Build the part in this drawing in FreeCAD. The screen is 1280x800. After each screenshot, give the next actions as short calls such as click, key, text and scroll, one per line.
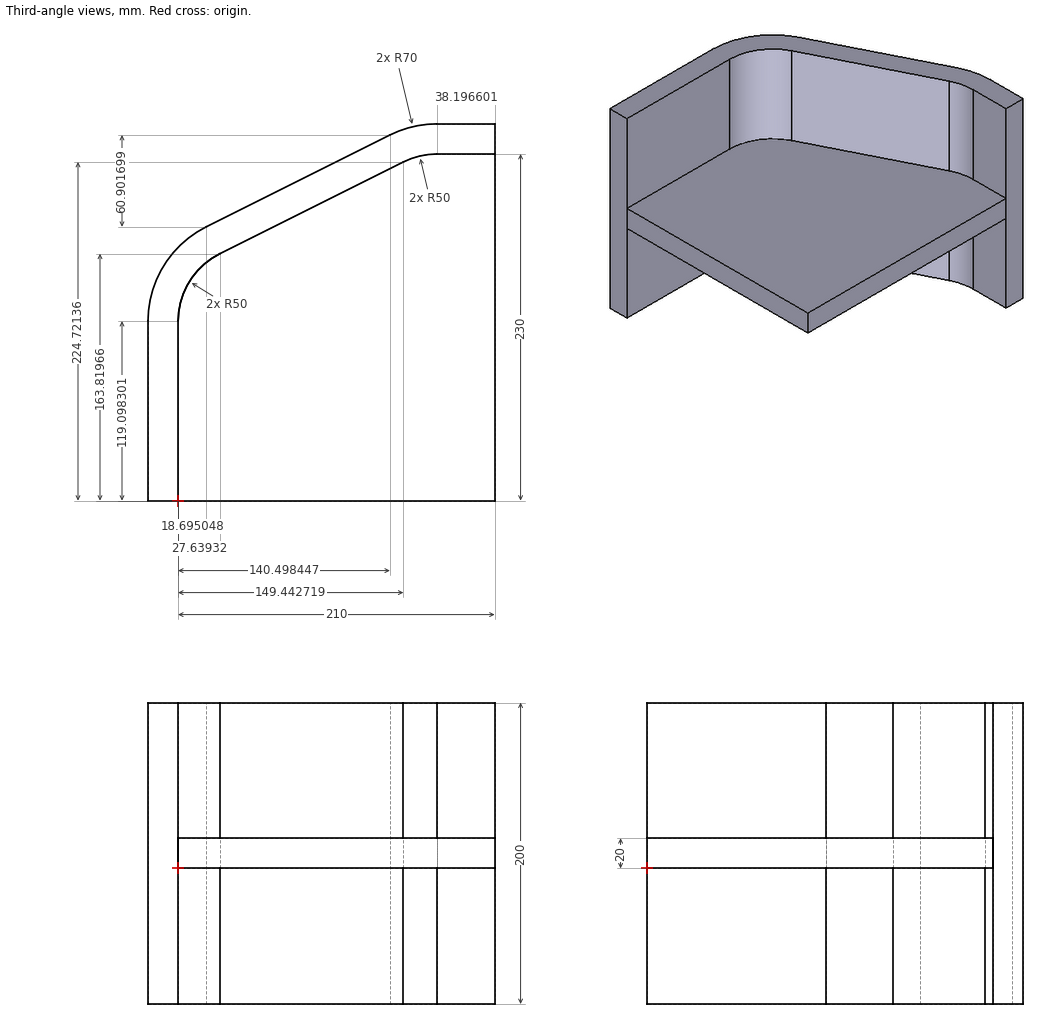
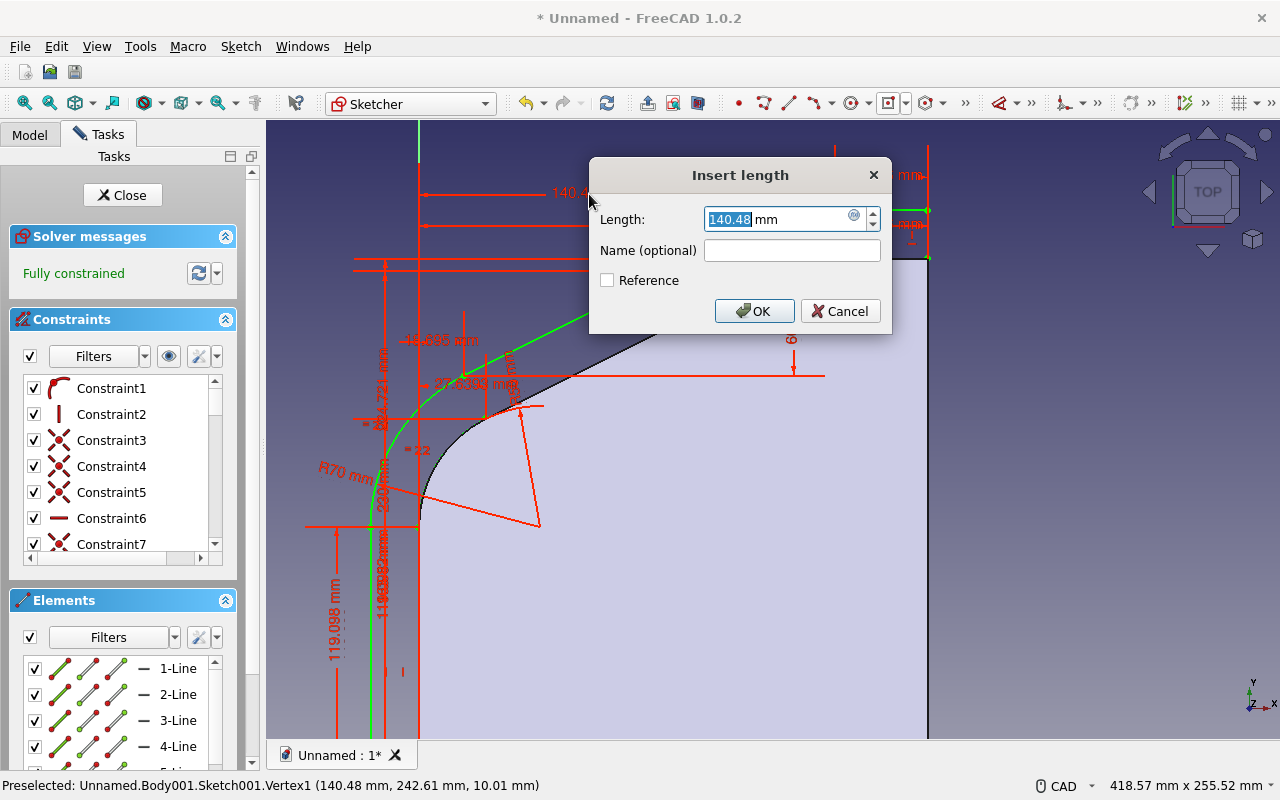
text(140.498447)
key(Return)
key(Escape)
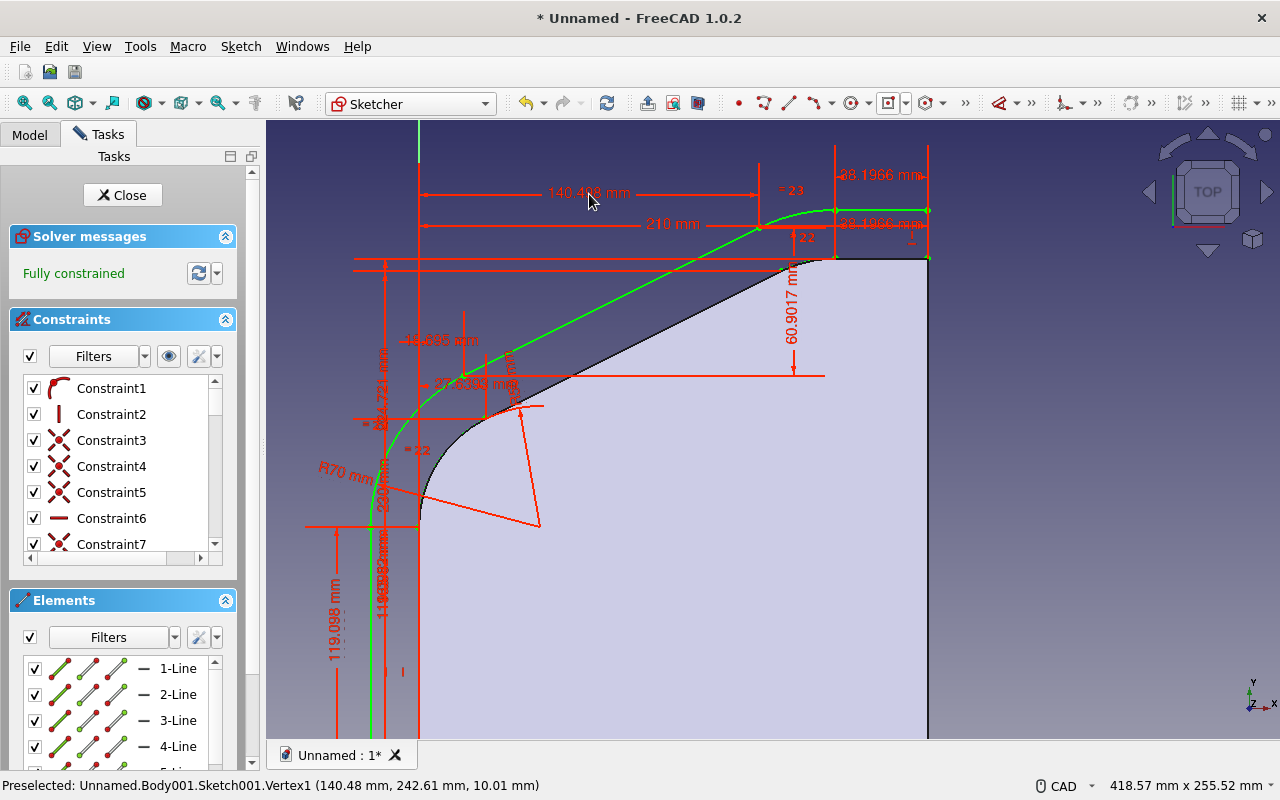
click(123, 195)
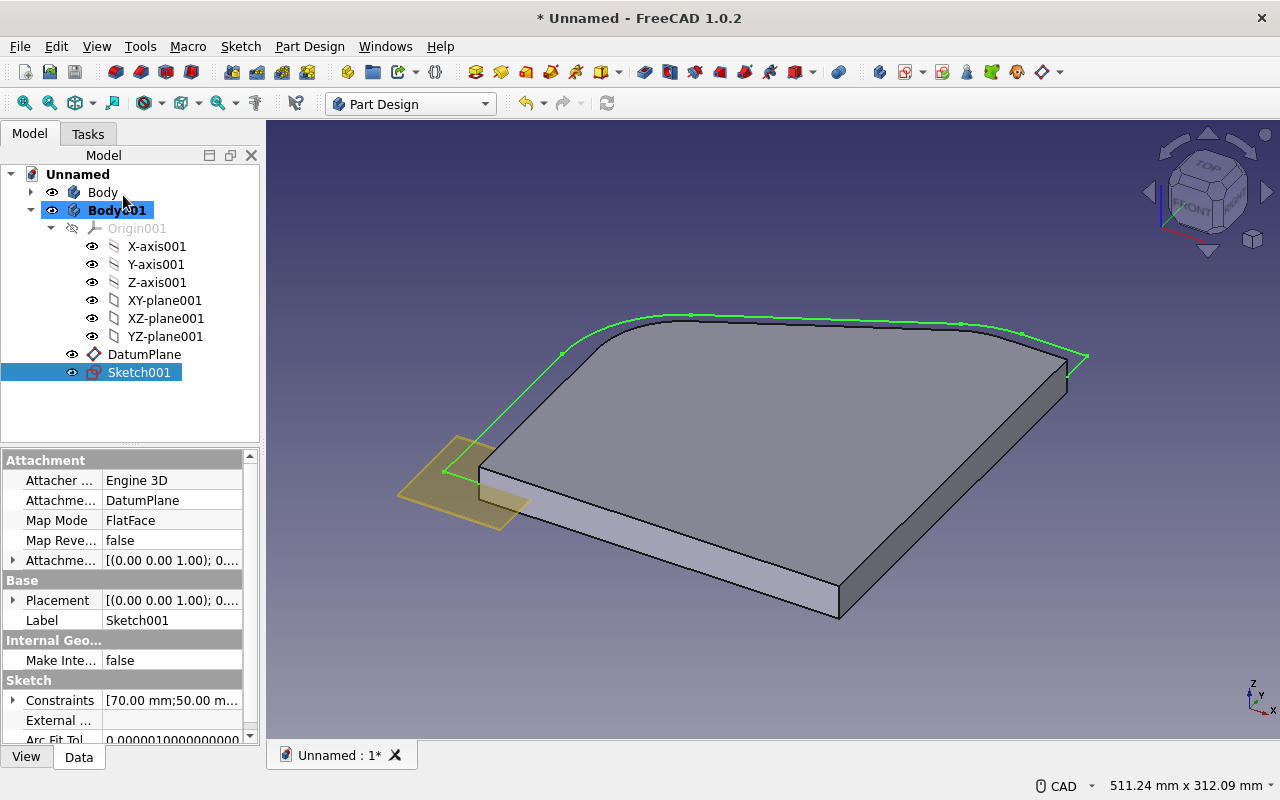
click(476, 72)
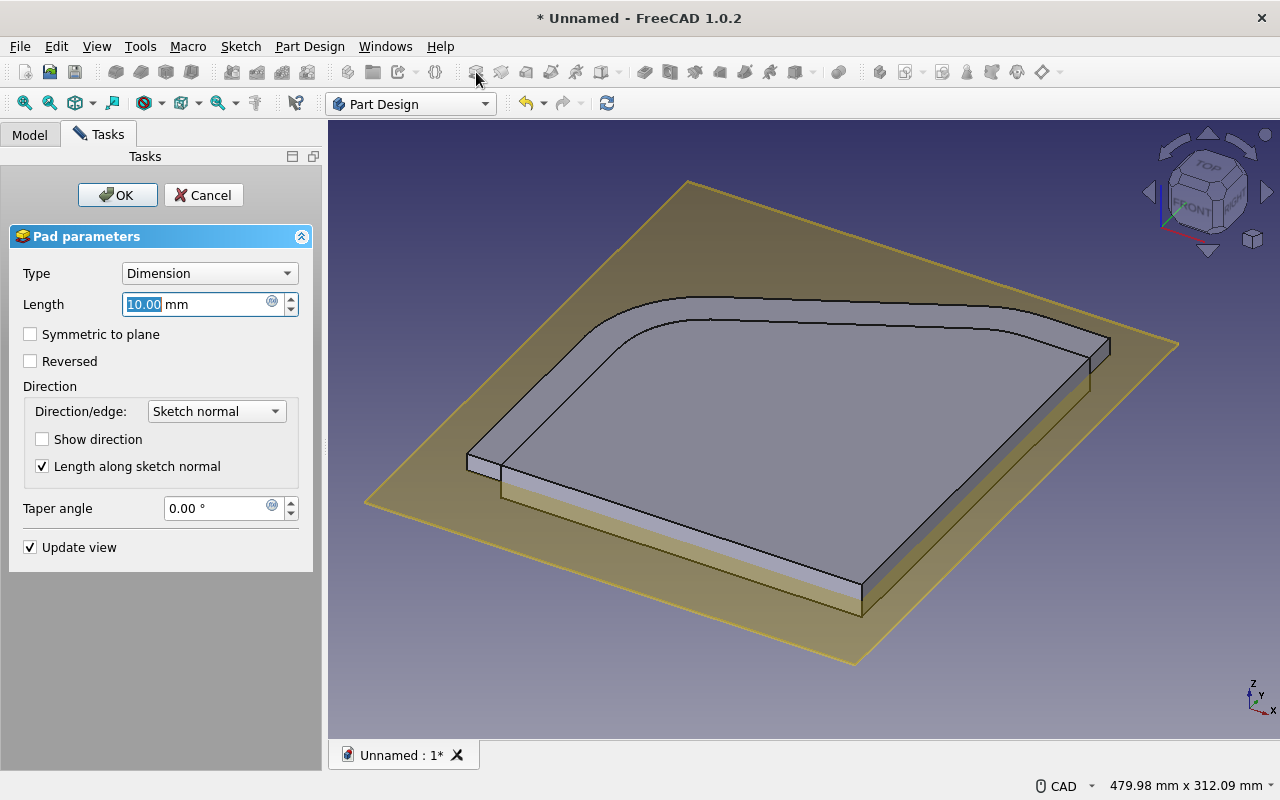
text(200)
key(Tab)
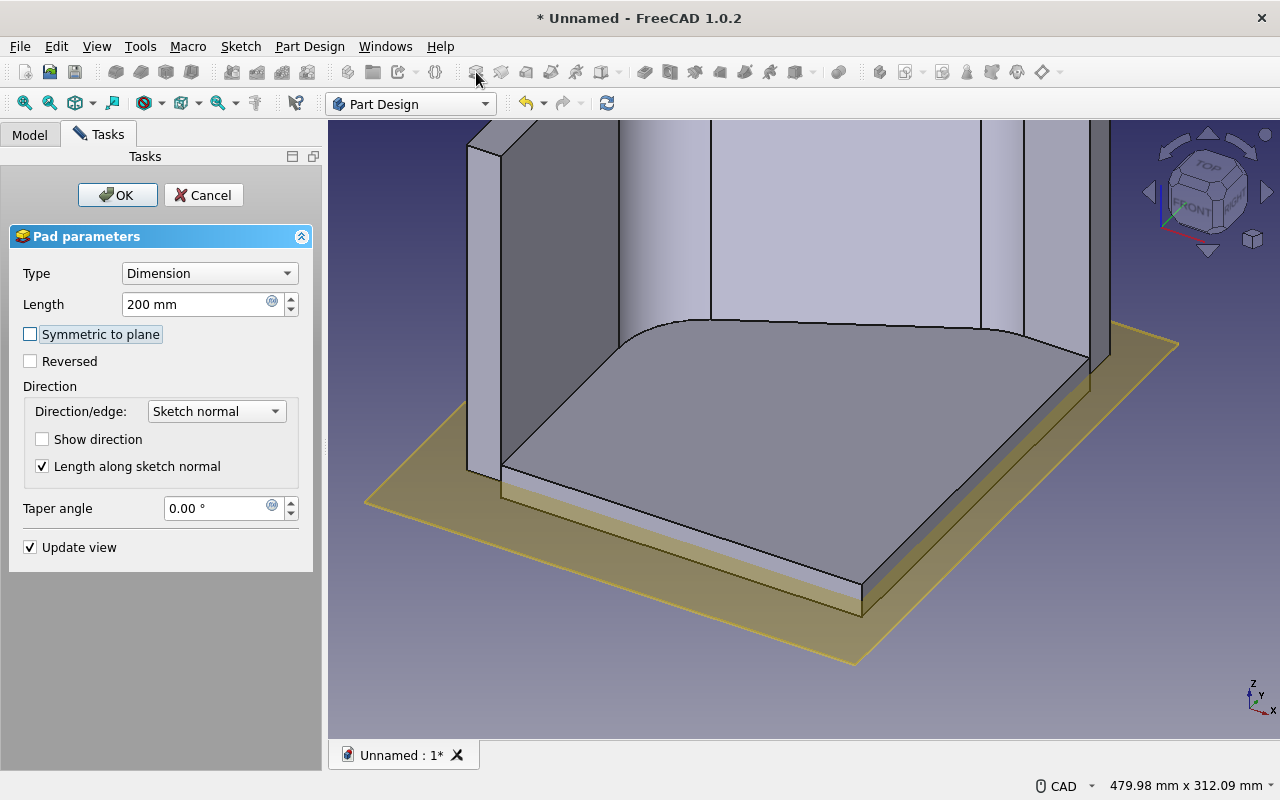
click(31, 334)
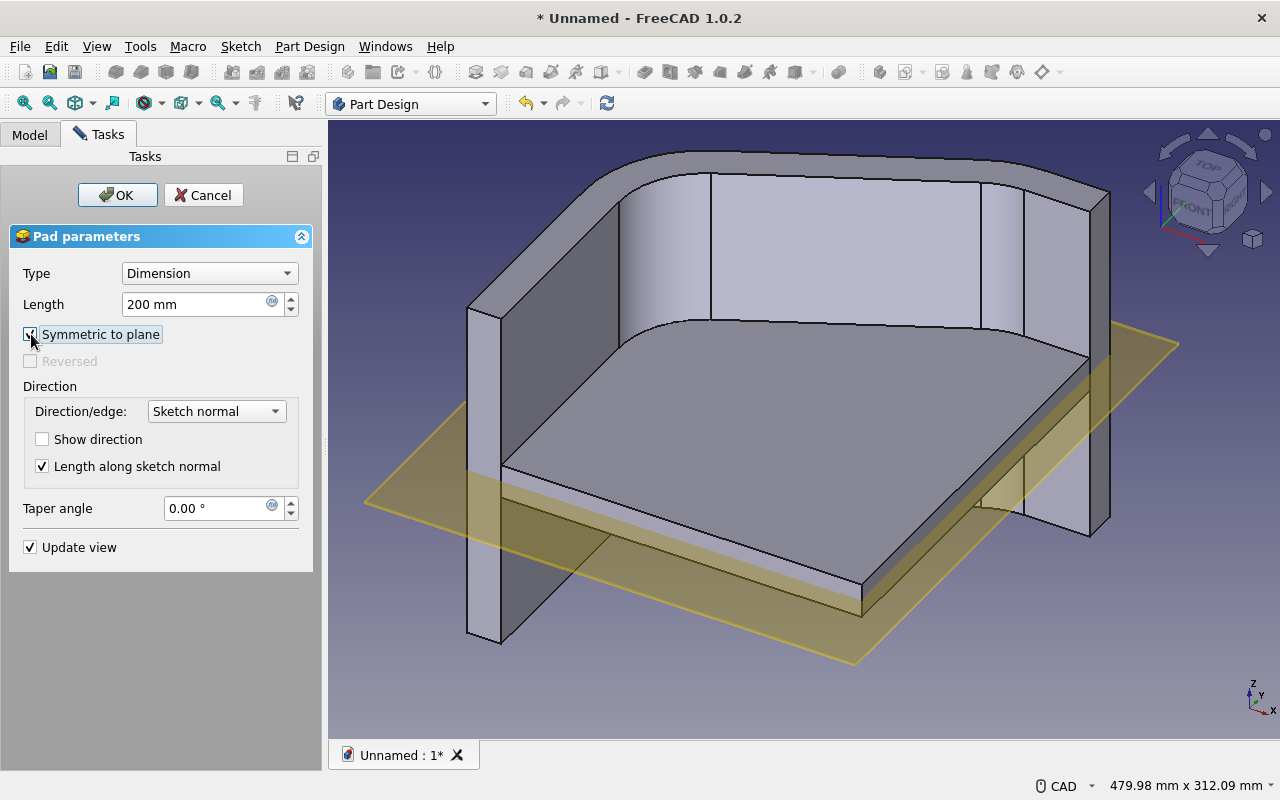
click(118, 195)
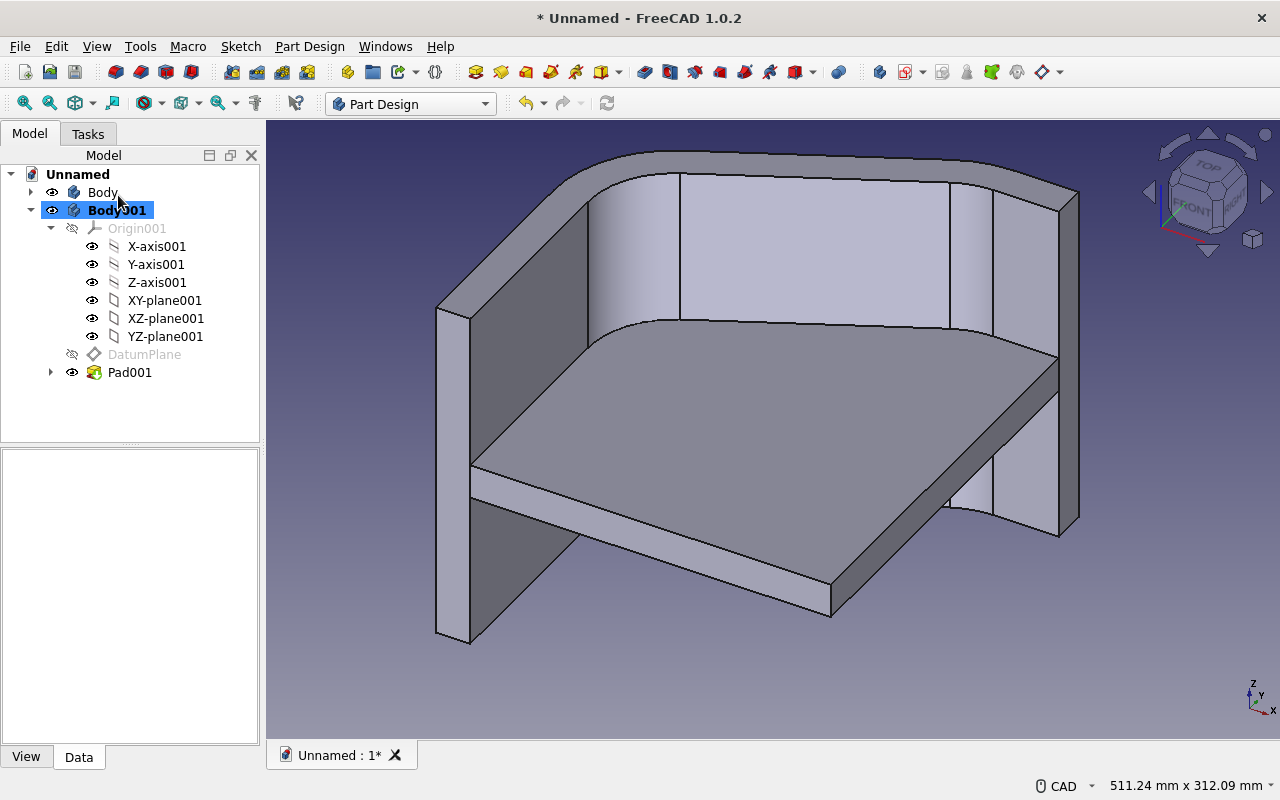
key(0)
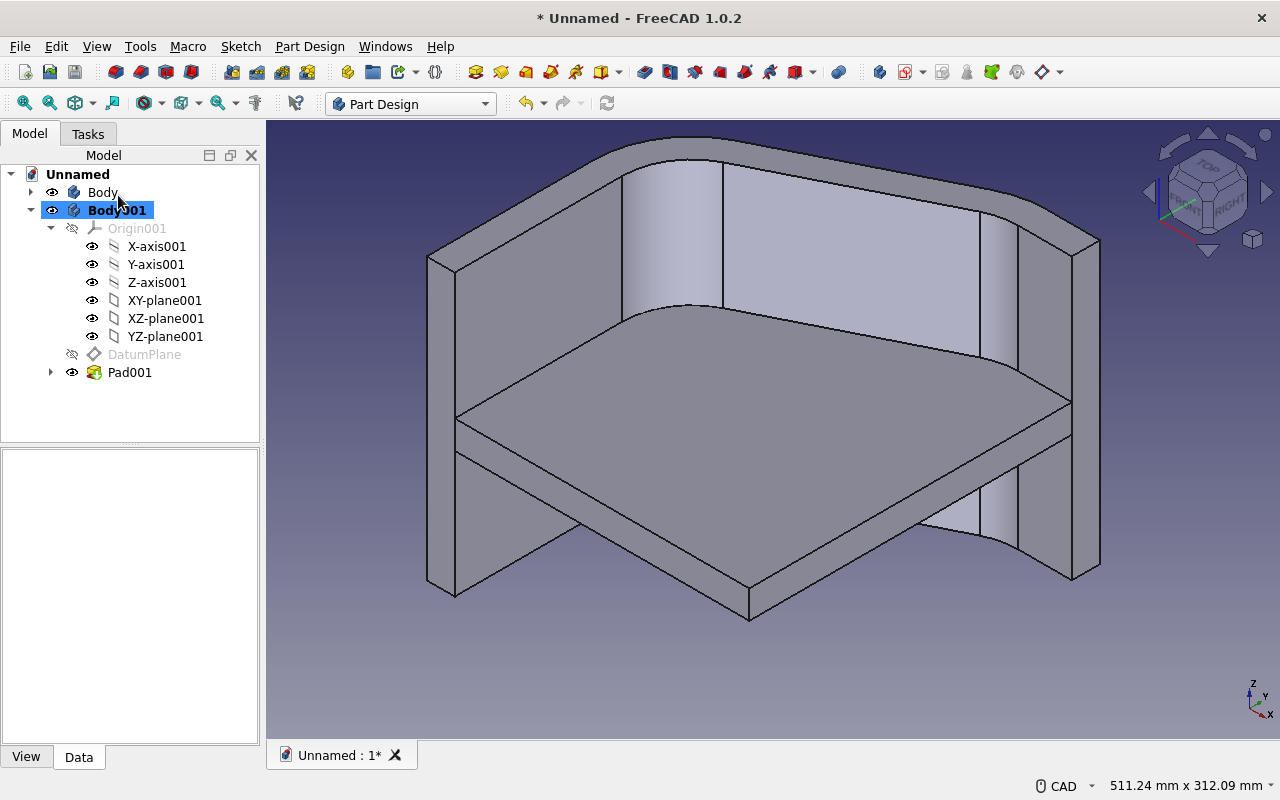
click(25, 104)